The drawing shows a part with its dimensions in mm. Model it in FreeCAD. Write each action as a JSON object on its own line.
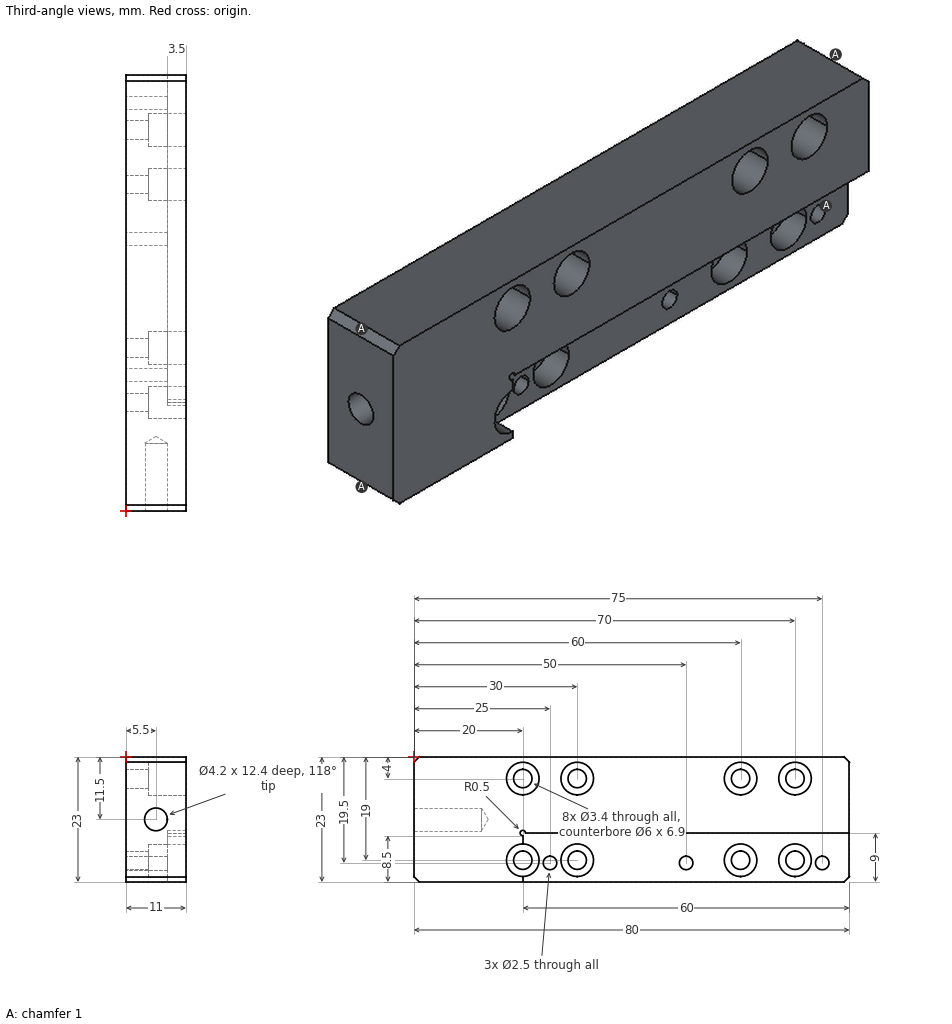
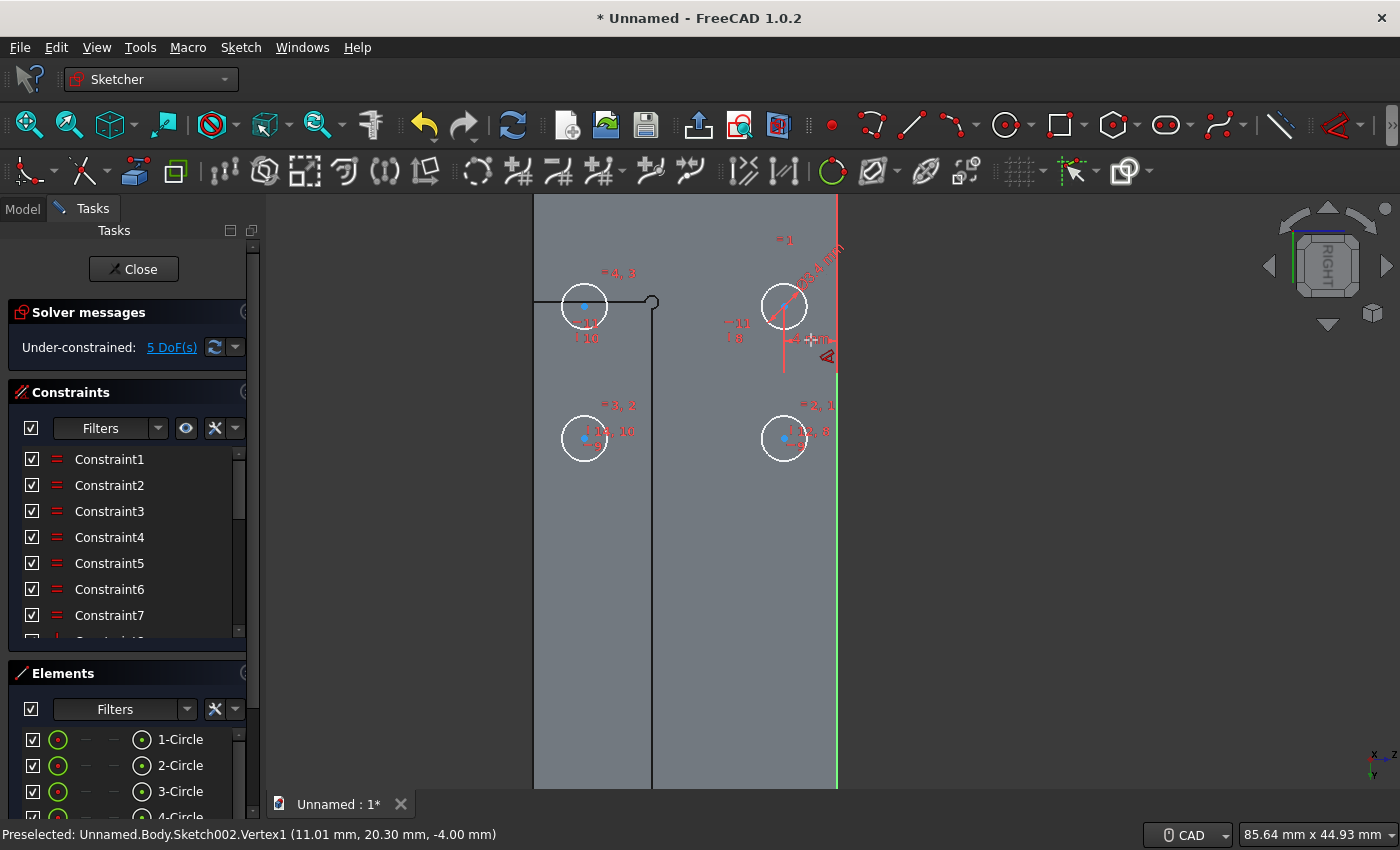
{"action": "left_click", "coordinate": [784, 306]}
{"action": "left_click", "coordinate": [871, 245]}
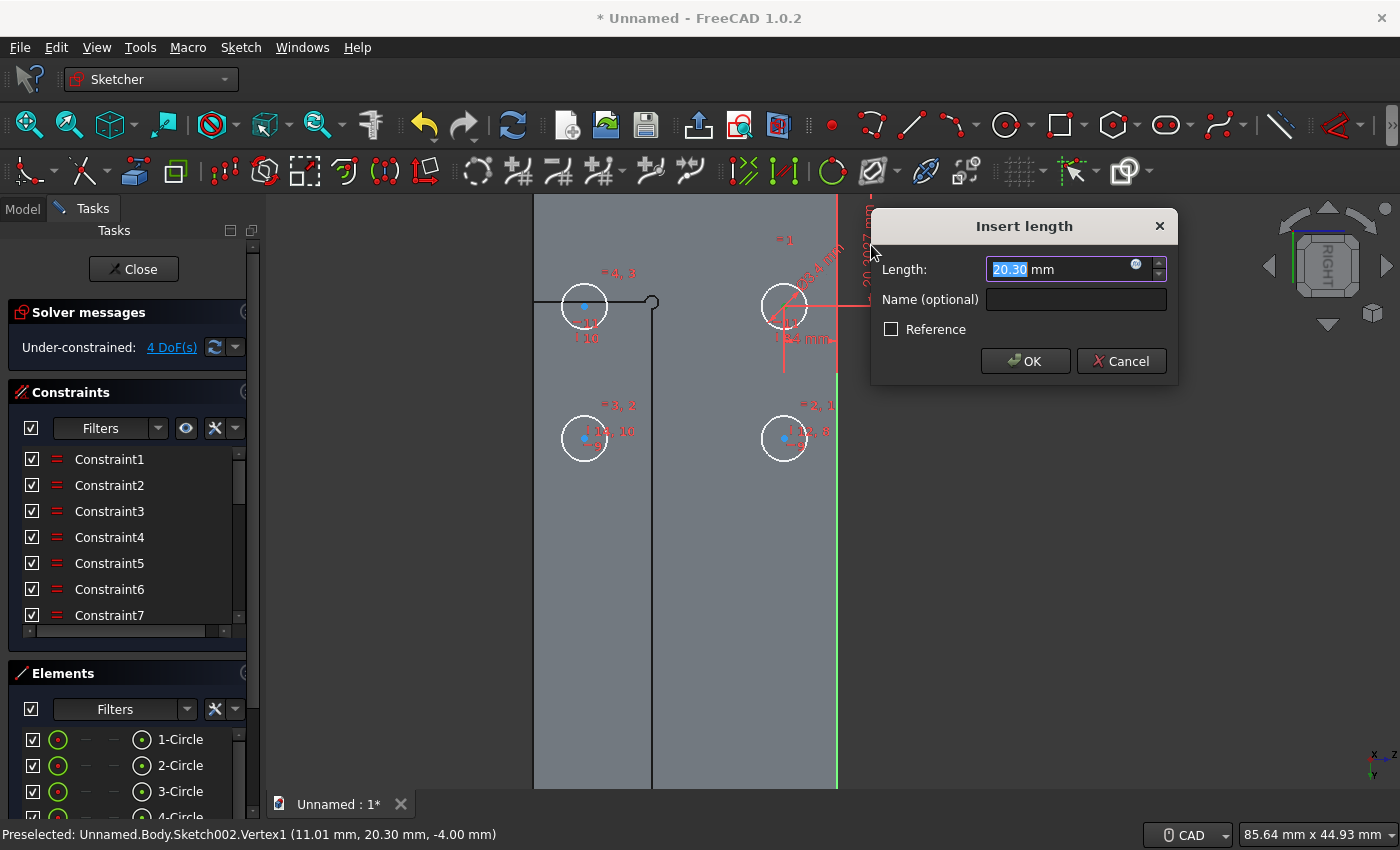
{"action": "type", "text": "20"}
{"action": "key", "text": "Return"}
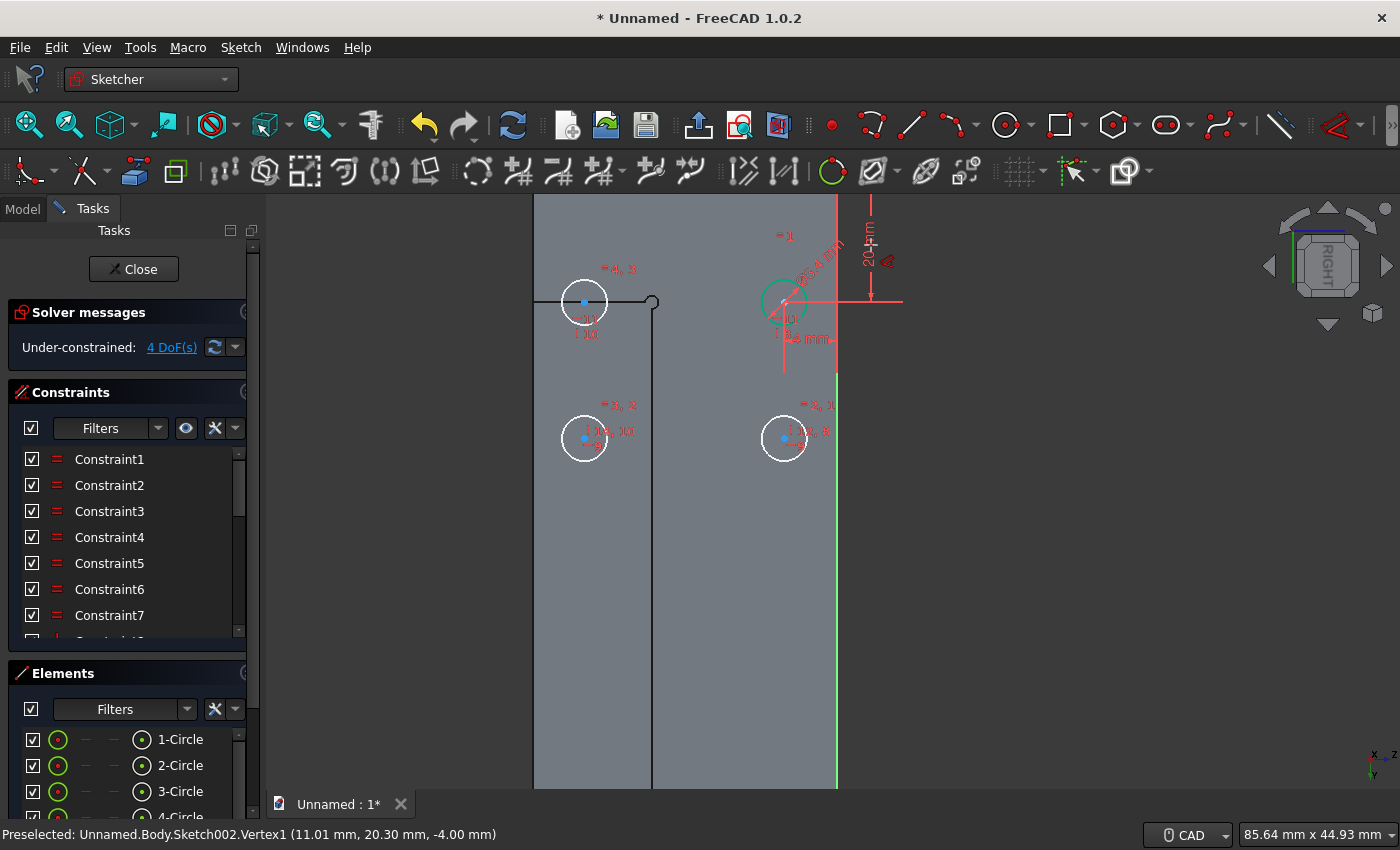
{"action": "left_click", "coordinate": [784, 439]}
{"action": "left_click", "coordinate": [871, 380]}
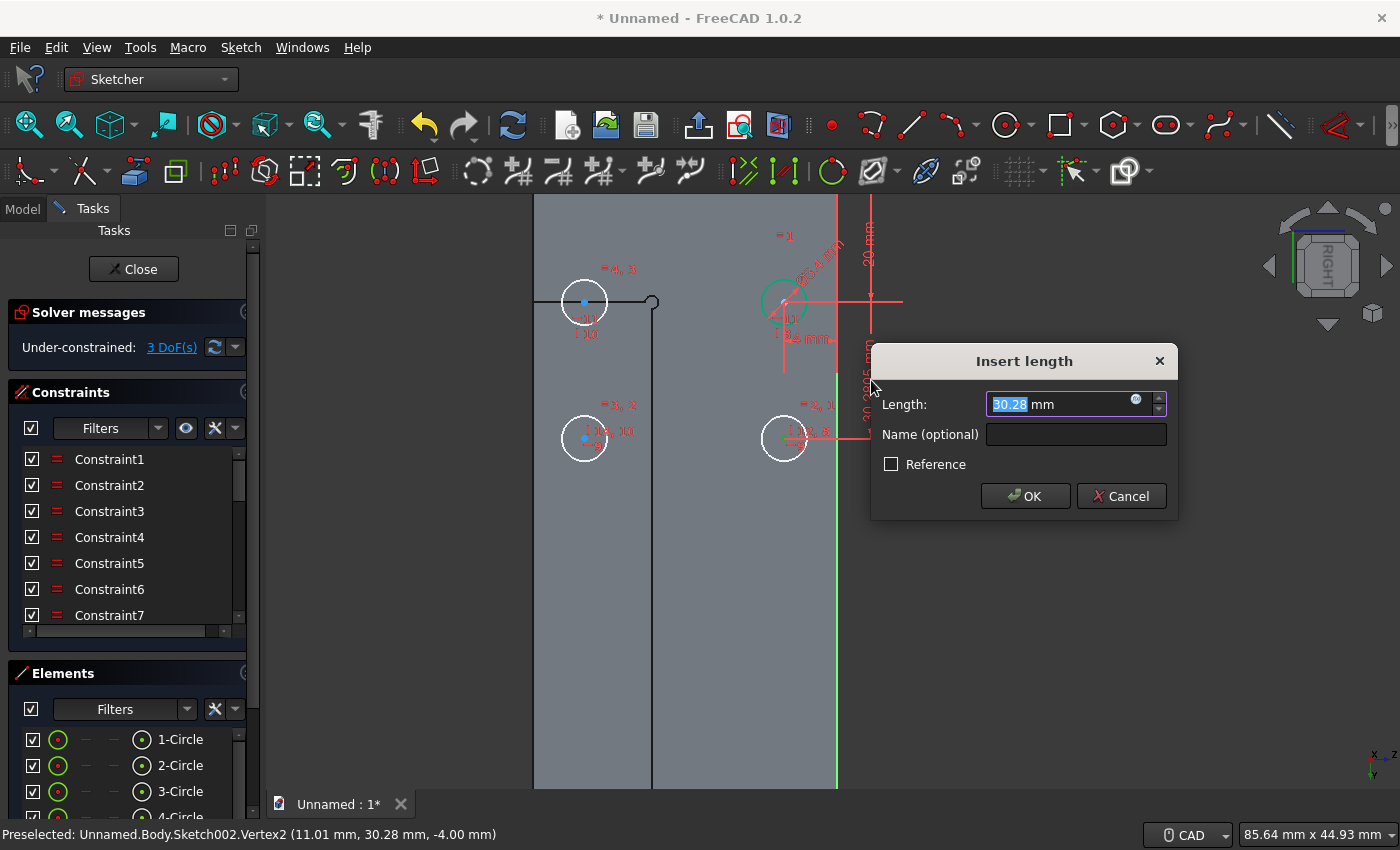
{"action": "type", "text": "30"}
{"action": "key", "text": "Return"}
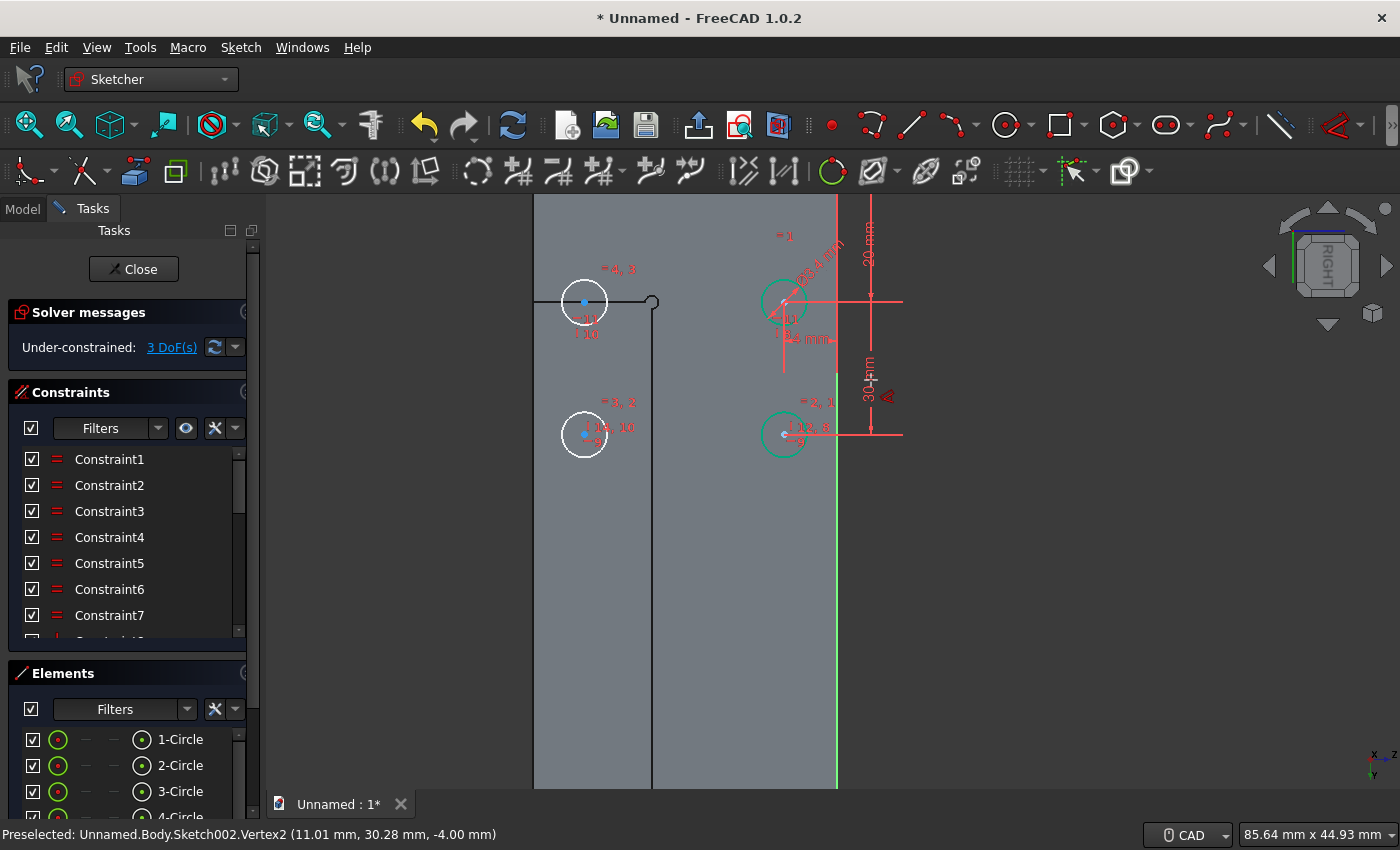
{"action": "left_click", "coordinate": [585, 435]}
{"action": "left_click", "coordinate": [711, 469]}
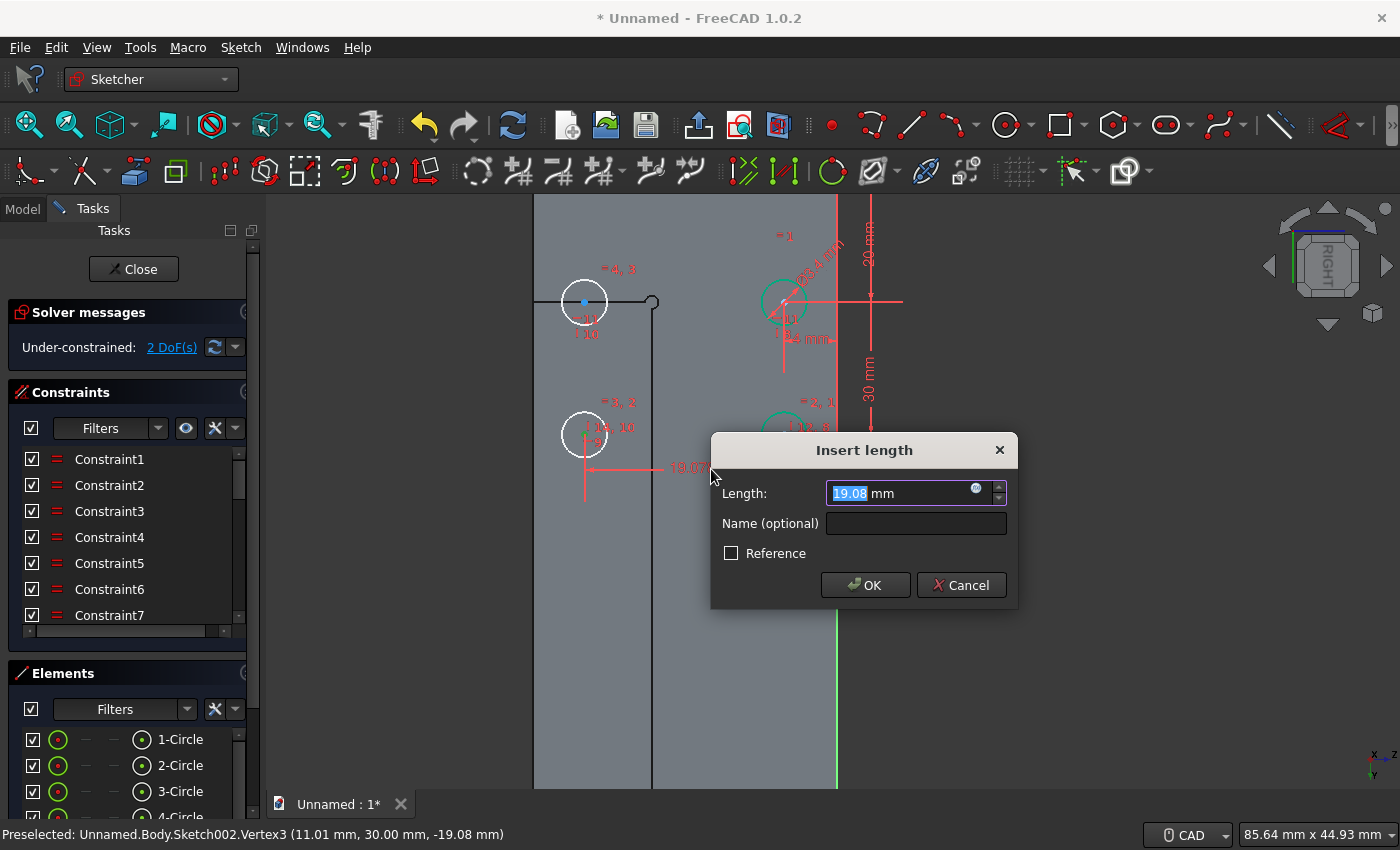
{"action": "type", "text": "19"}
{"action": "key", "text": "Return"}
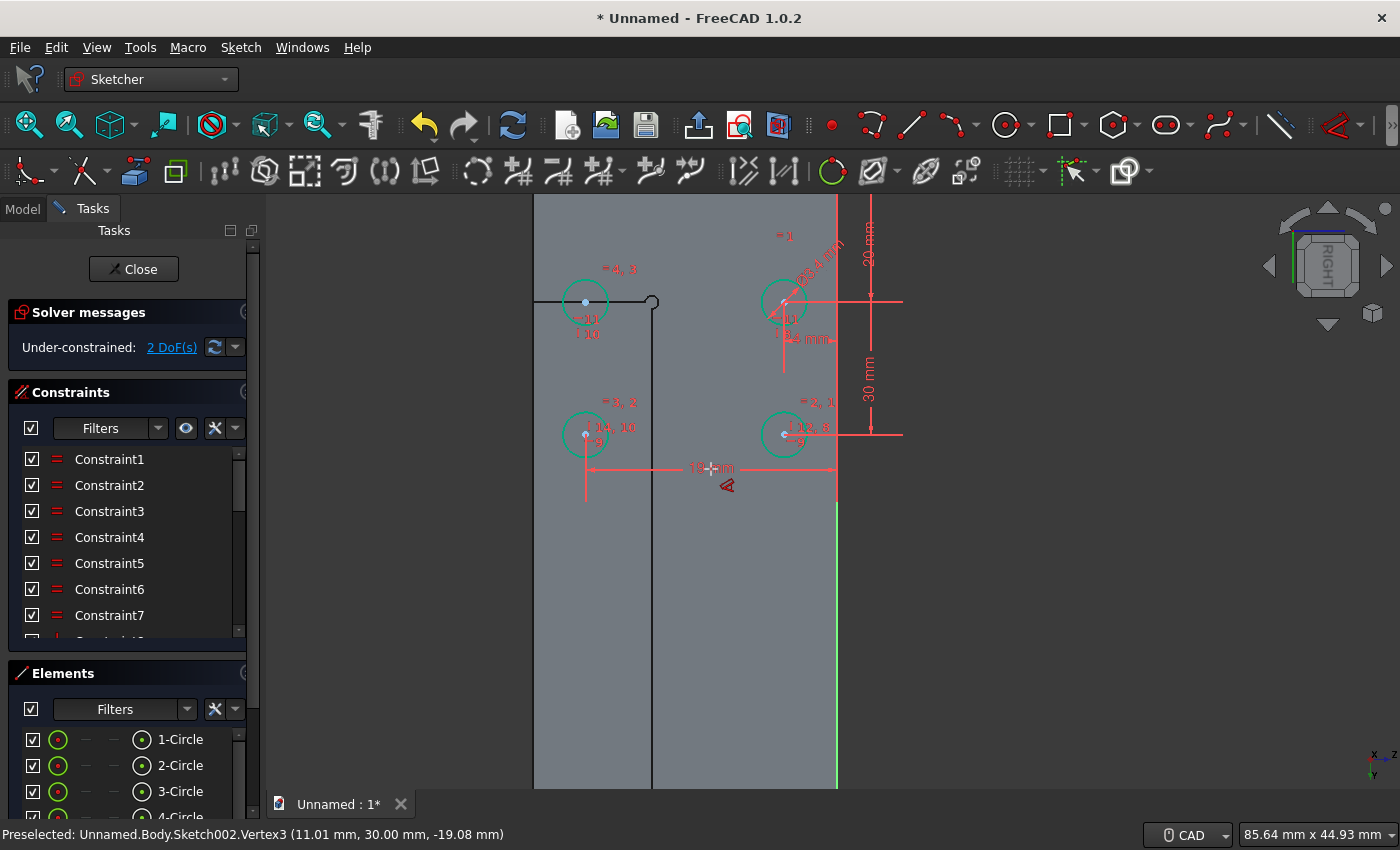
{"action": "scroll", "coordinate": [802, 479], "scroll_direction": "down", "scroll_amount": 5}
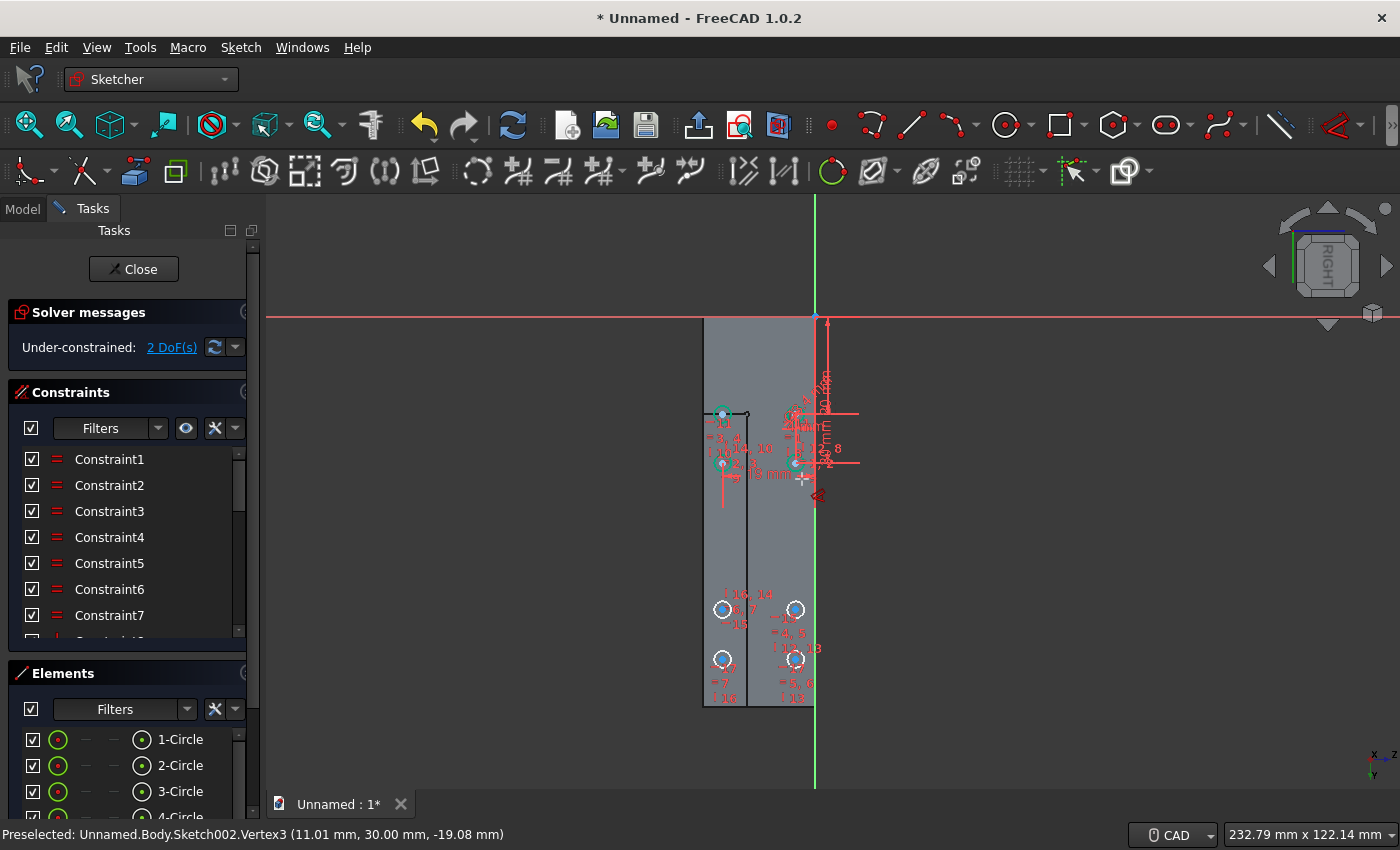
{"action": "left_click", "coordinate": [796, 610]}
{"action": "left_click", "coordinate": [849, 463]}